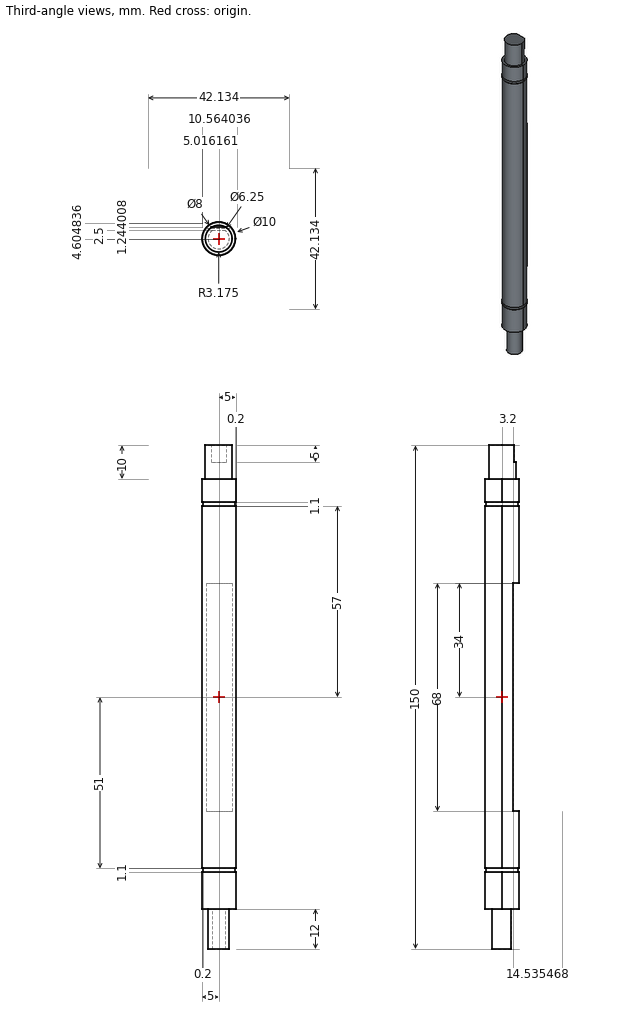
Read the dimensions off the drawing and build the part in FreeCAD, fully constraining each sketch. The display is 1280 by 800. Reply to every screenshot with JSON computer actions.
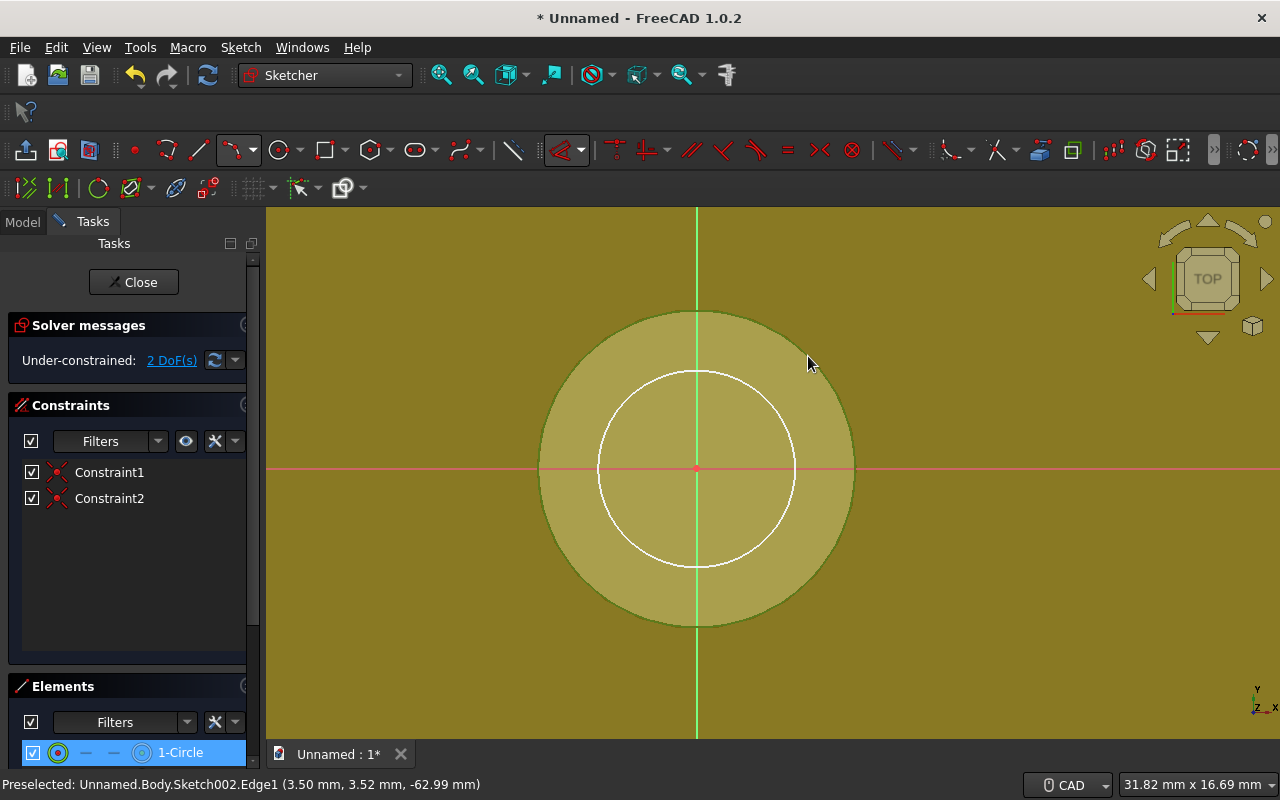
{"action": "left_click", "coordinate": [584, 150]}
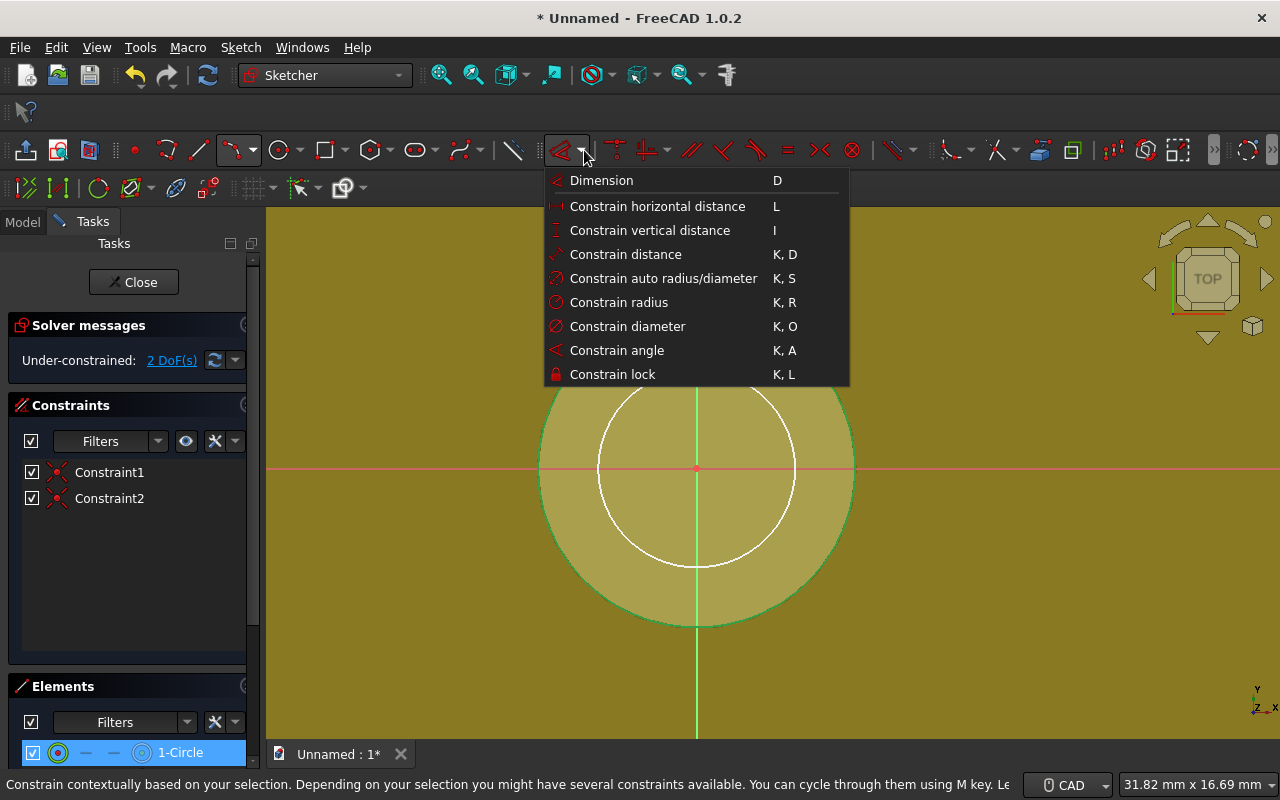
{"action": "left_click", "coordinate": [697, 326]}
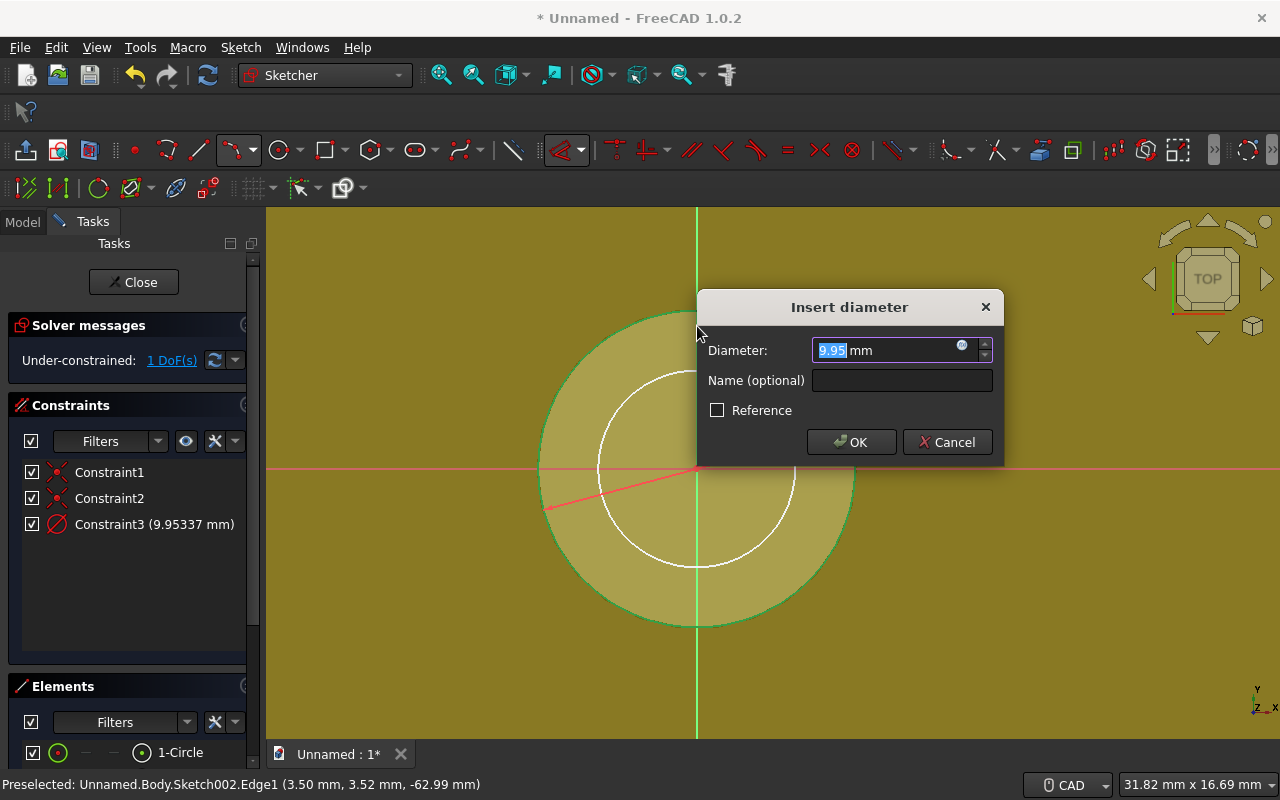
{"action": "type", "text": "10"}
{"action": "key", "text": "Return"}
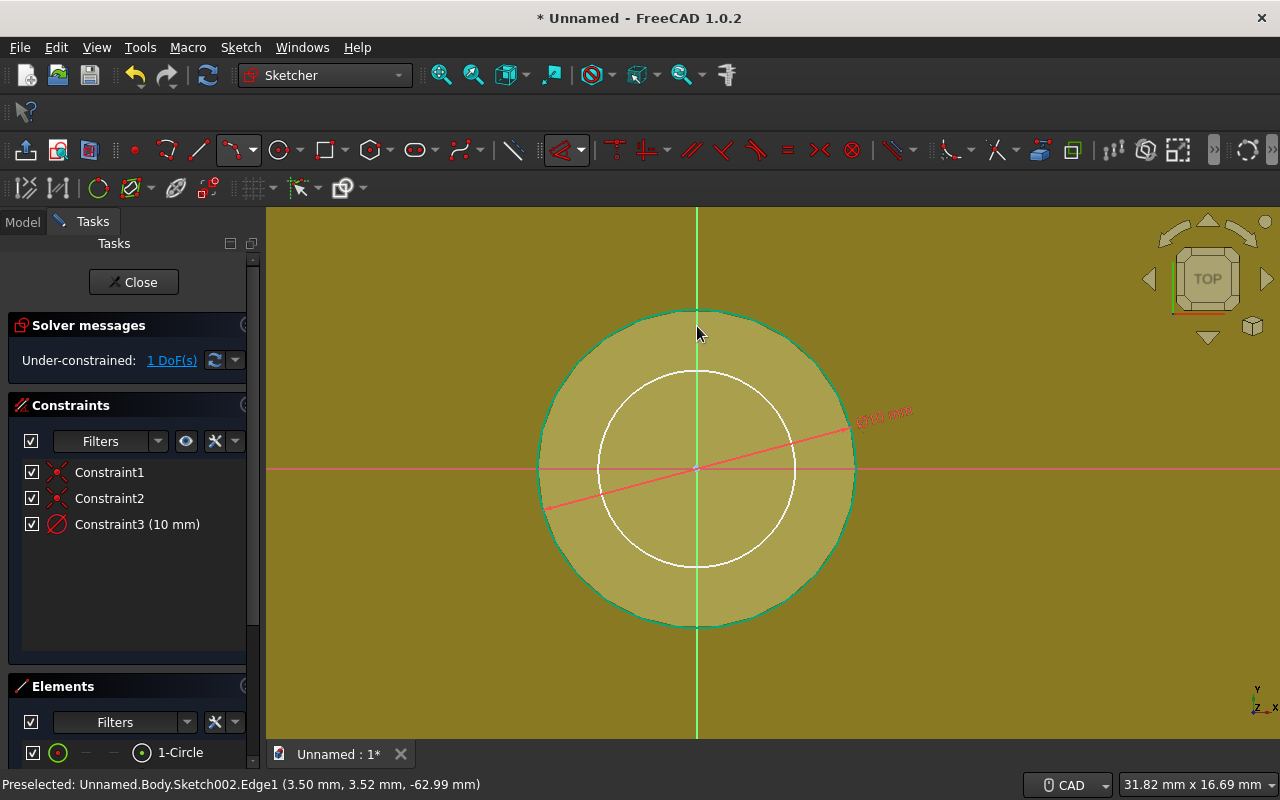
{"action": "left_click", "coordinate": [766, 399]}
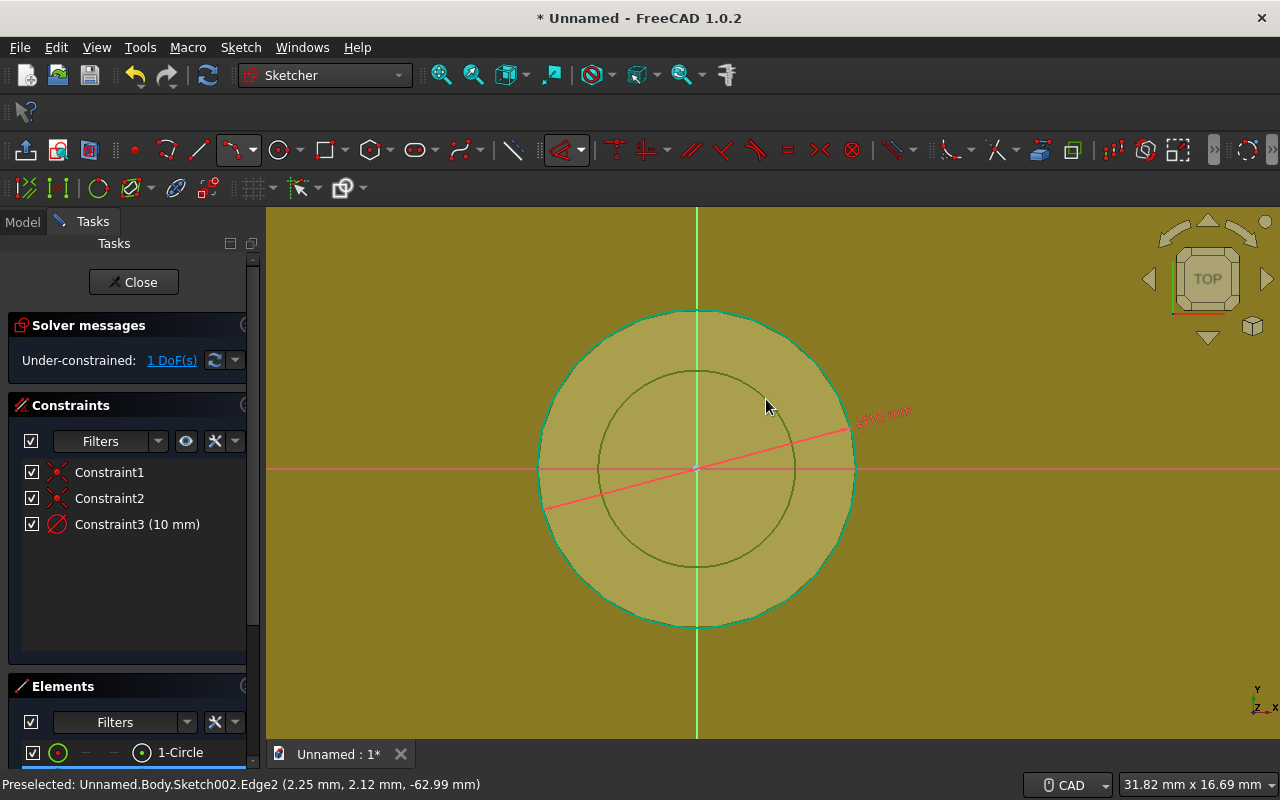
{"action": "left_click", "coordinate": [584, 150]}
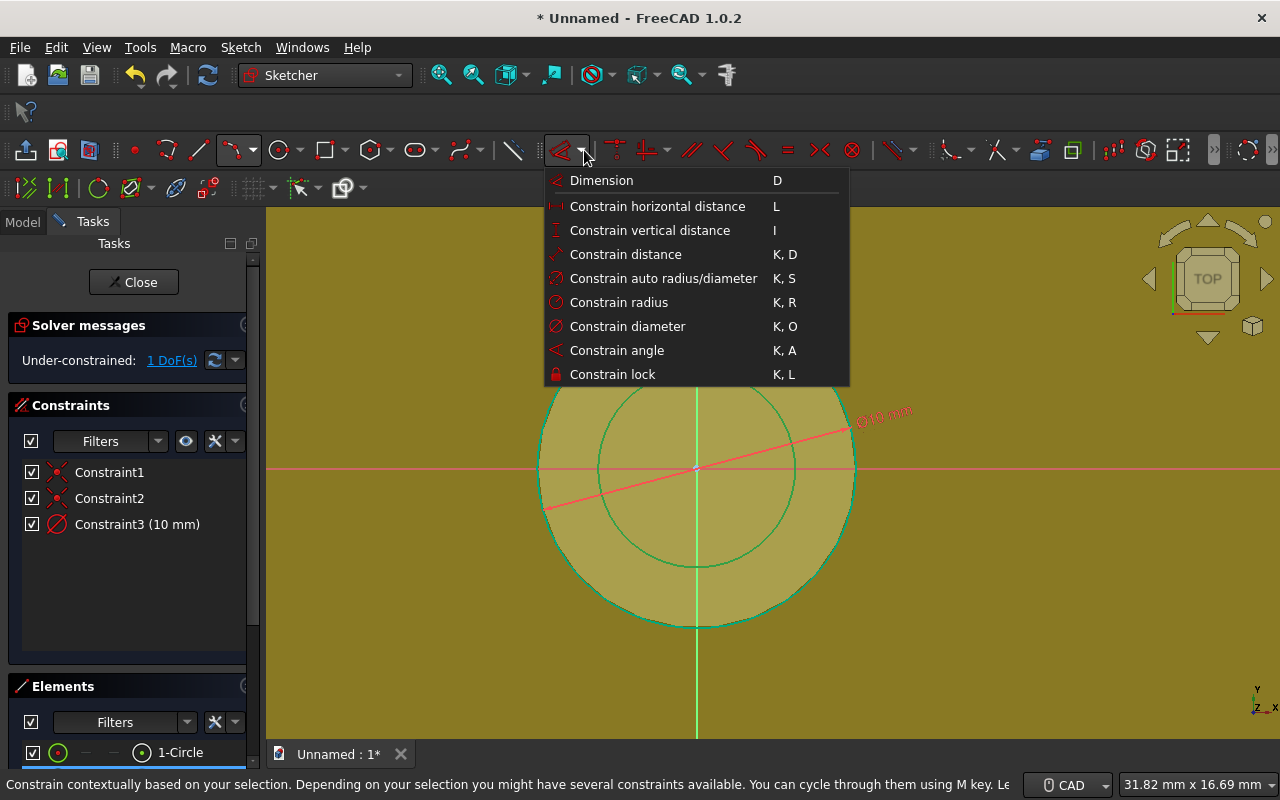
{"action": "left_click", "coordinate": [697, 326]}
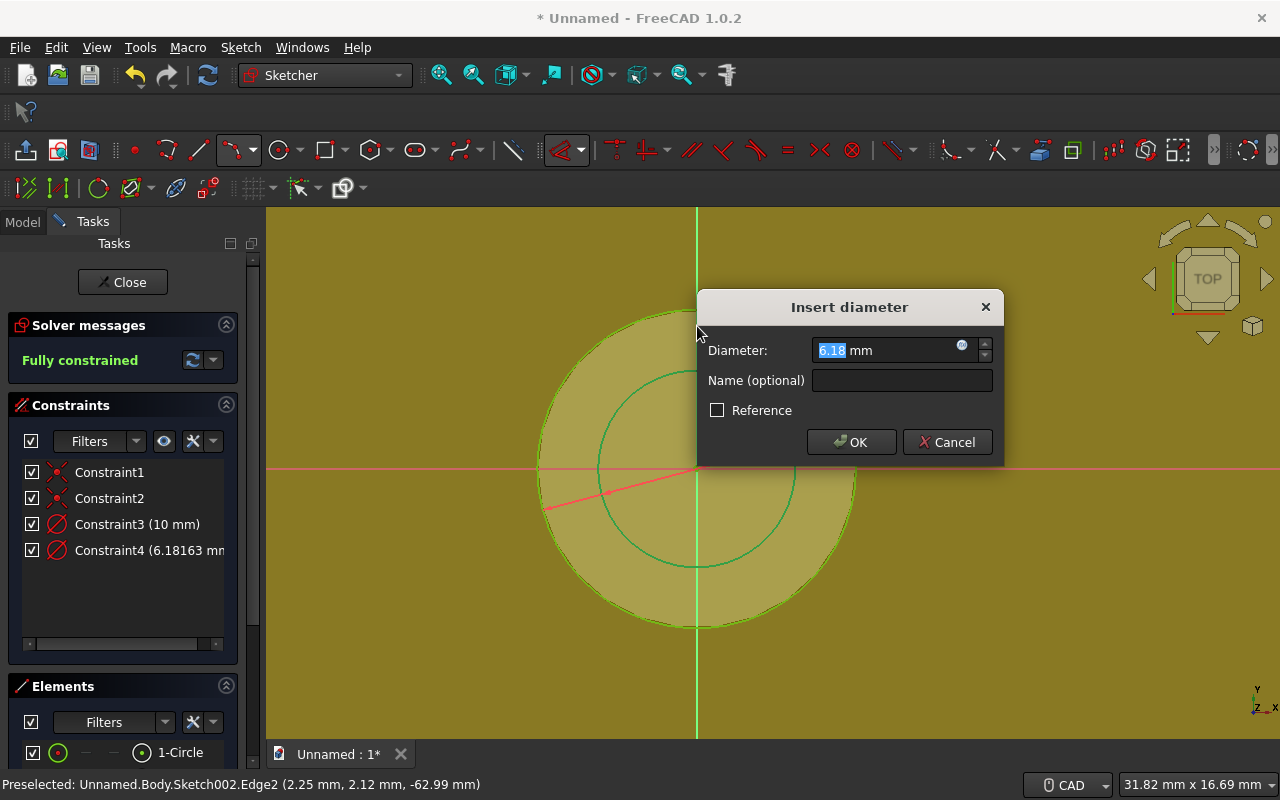
{"action": "type", "text": "6.25"}
{"action": "key", "text": "Return"}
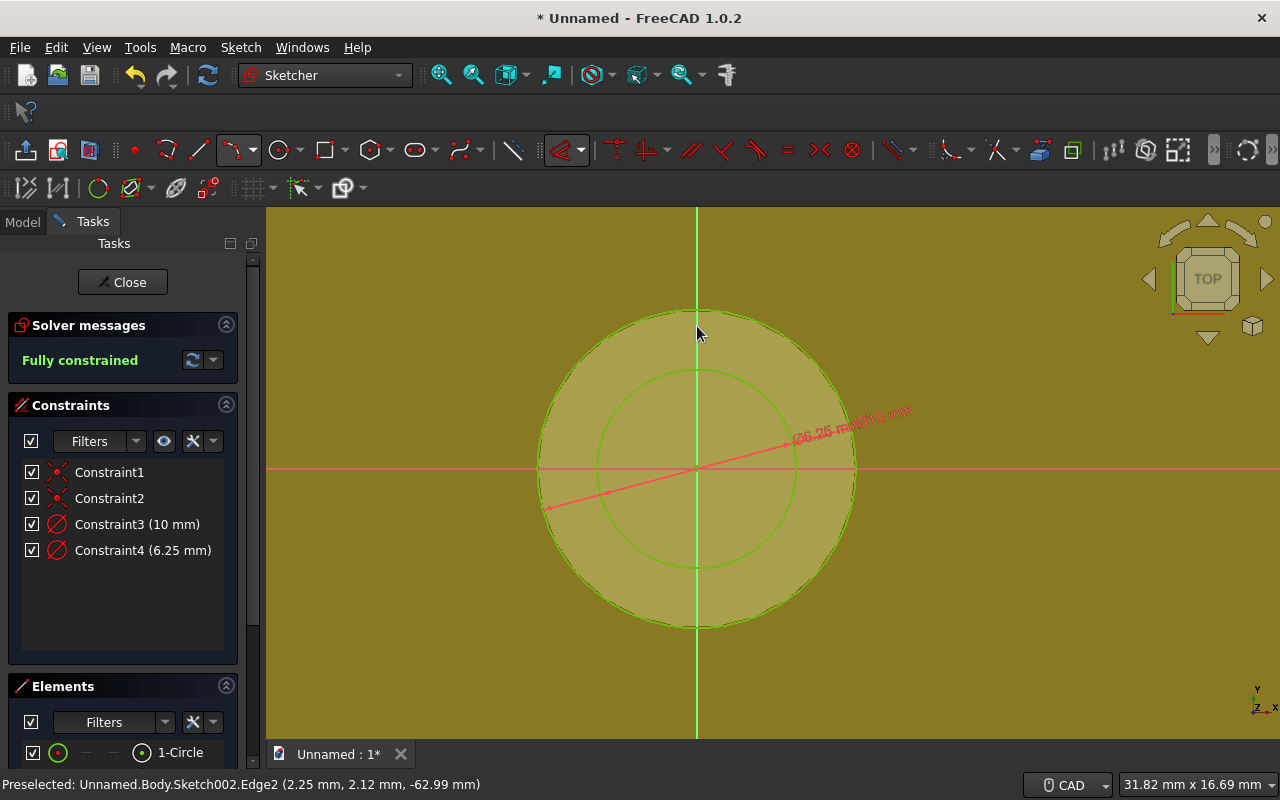
{"action": "left_click", "coordinate": [123, 282]}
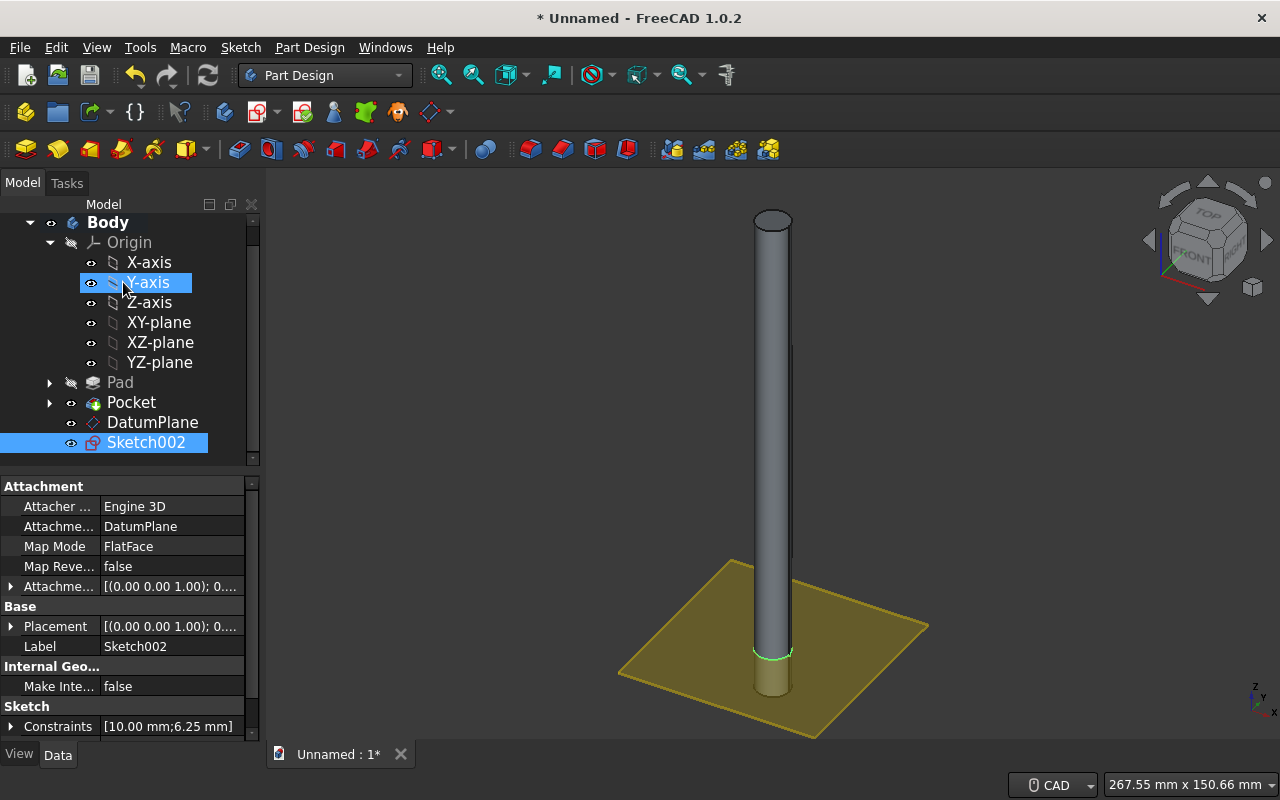
{"action": "left_click", "coordinate": [240, 150]}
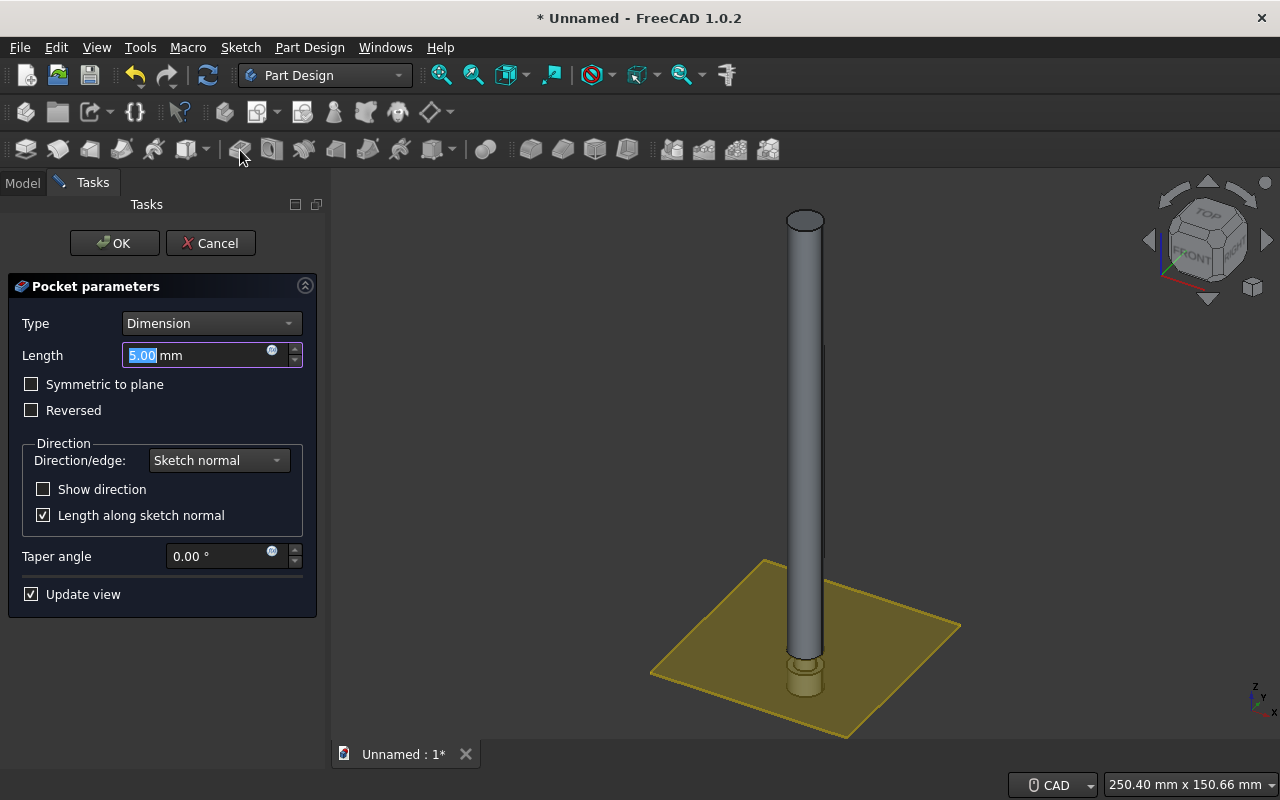
{"action": "type", "text": "12"}
{"action": "key", "text": "Tab"}